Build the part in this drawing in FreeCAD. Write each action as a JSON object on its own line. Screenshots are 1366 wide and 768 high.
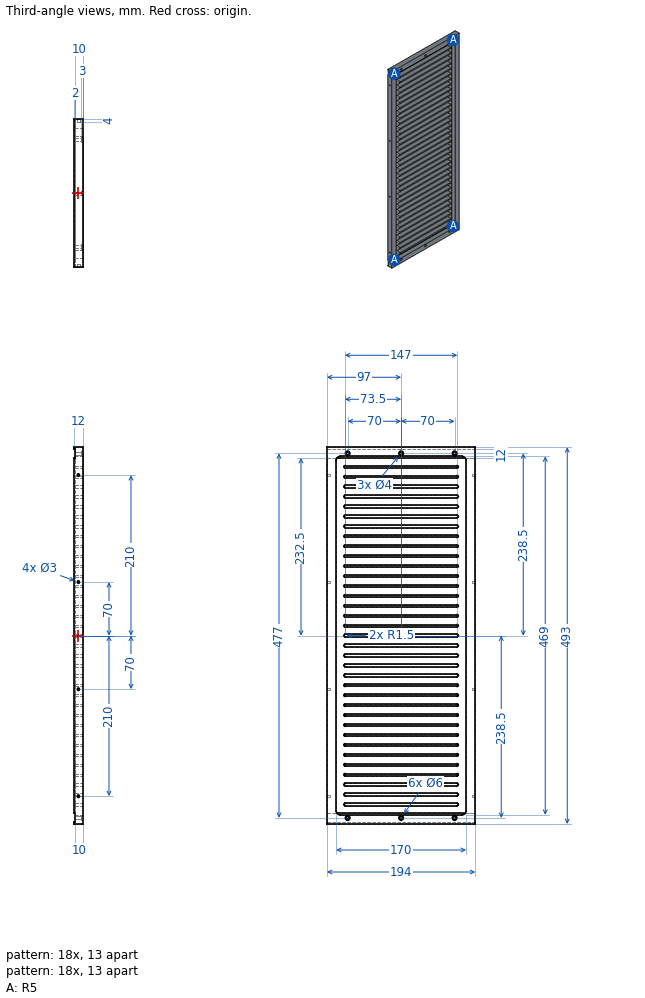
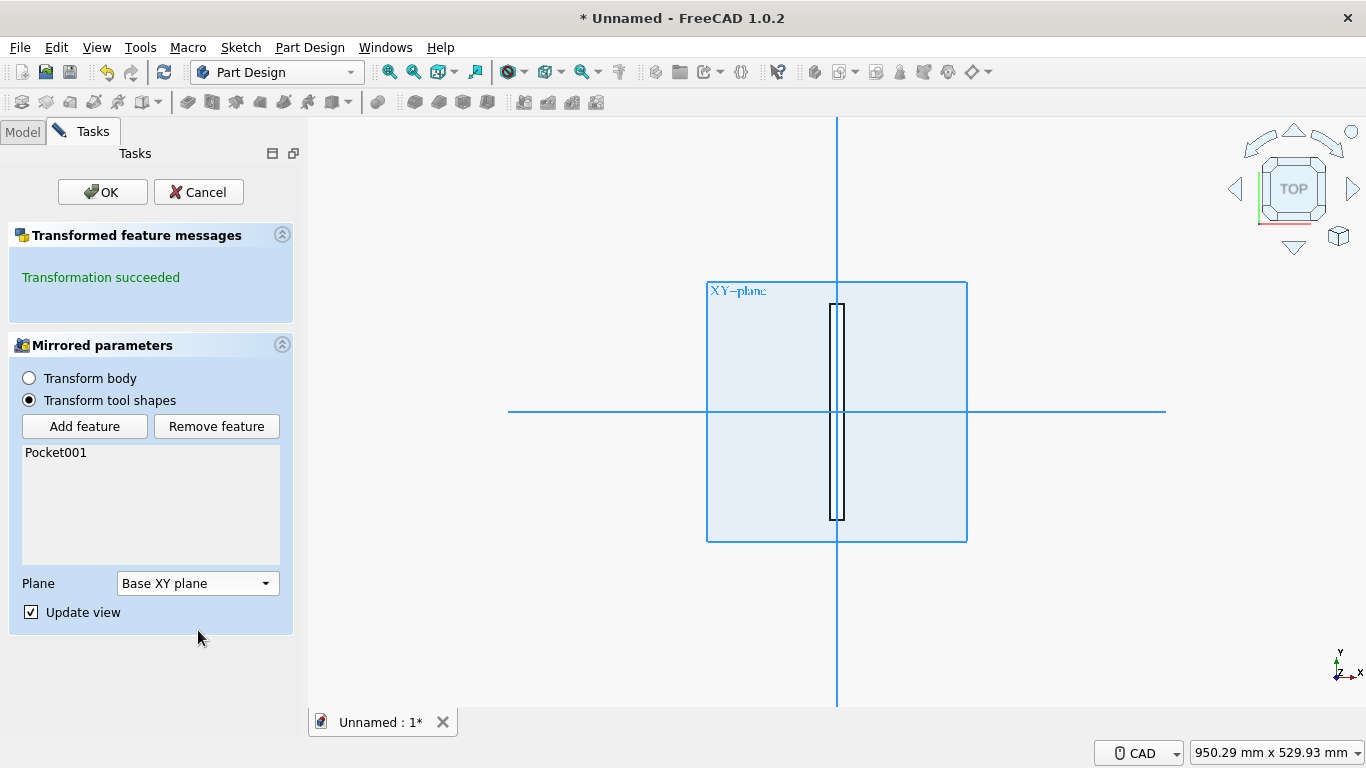
{"action": "left_click", "coordinate": [103, 192]}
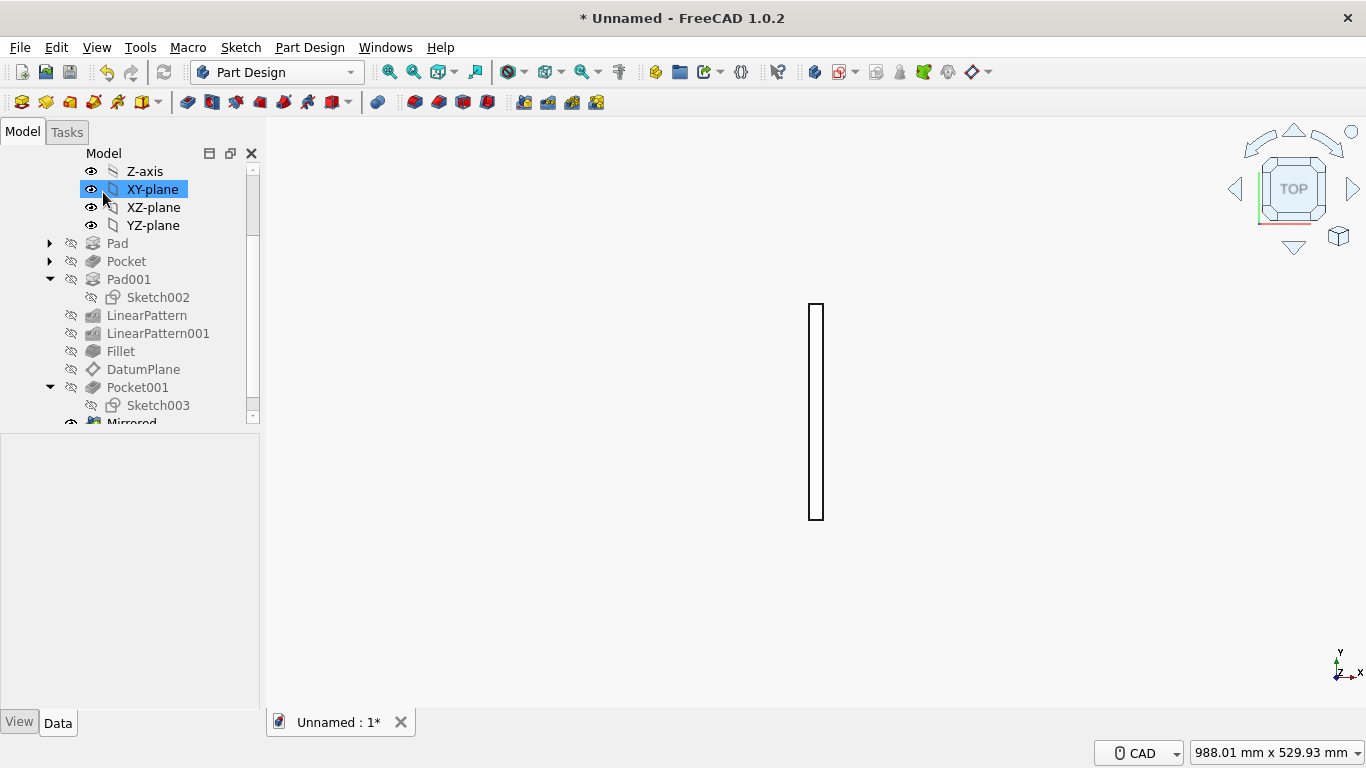
{"action": "left_click", "coordinate": [390, 72]}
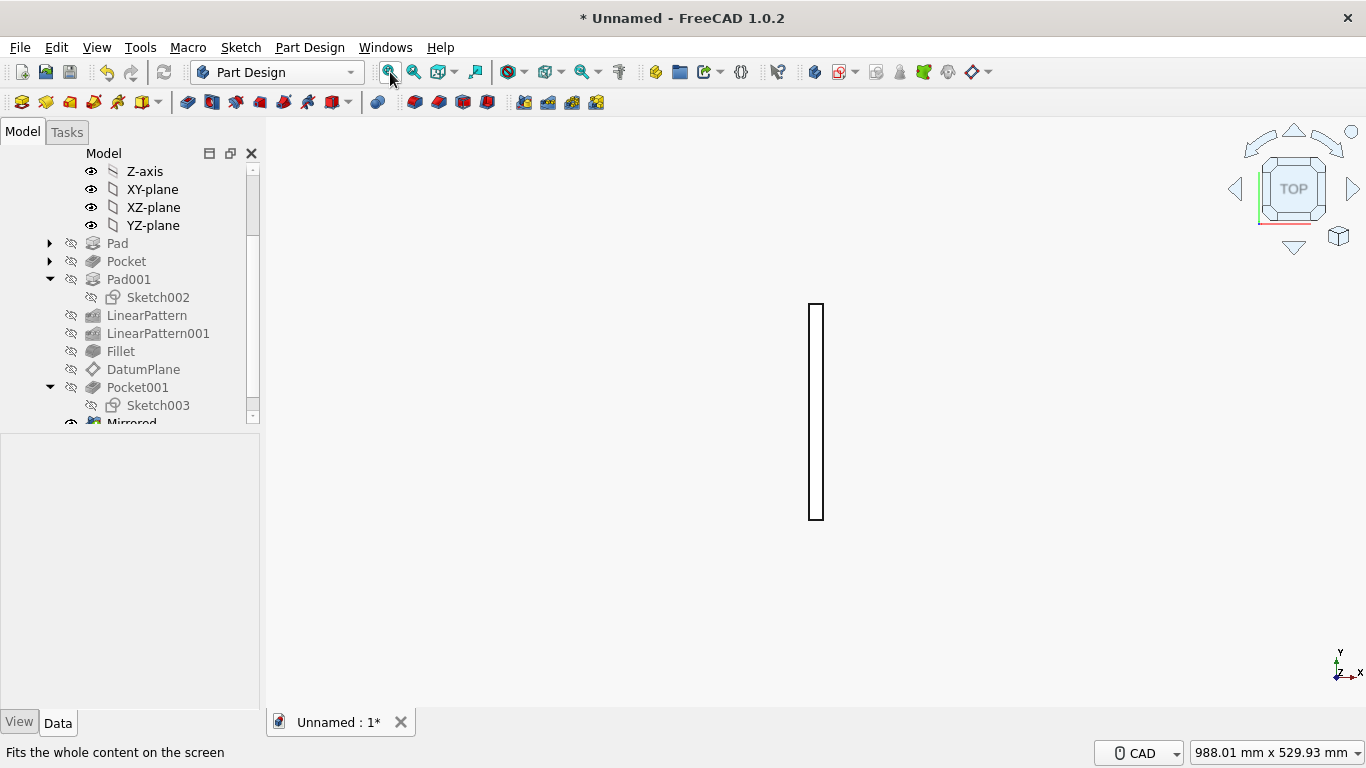
{"action": "key", "text": "6"}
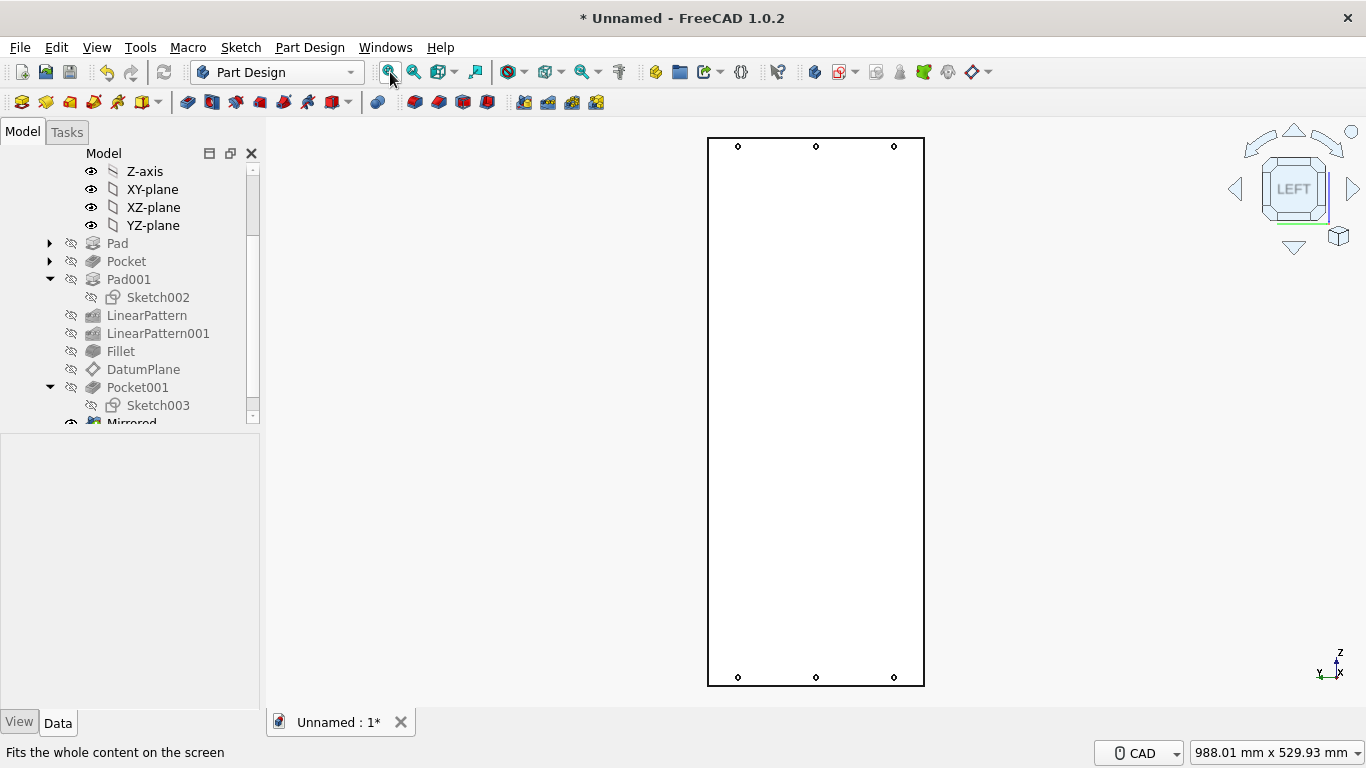
{"action": "left_click", "coordinate": [816, 489]}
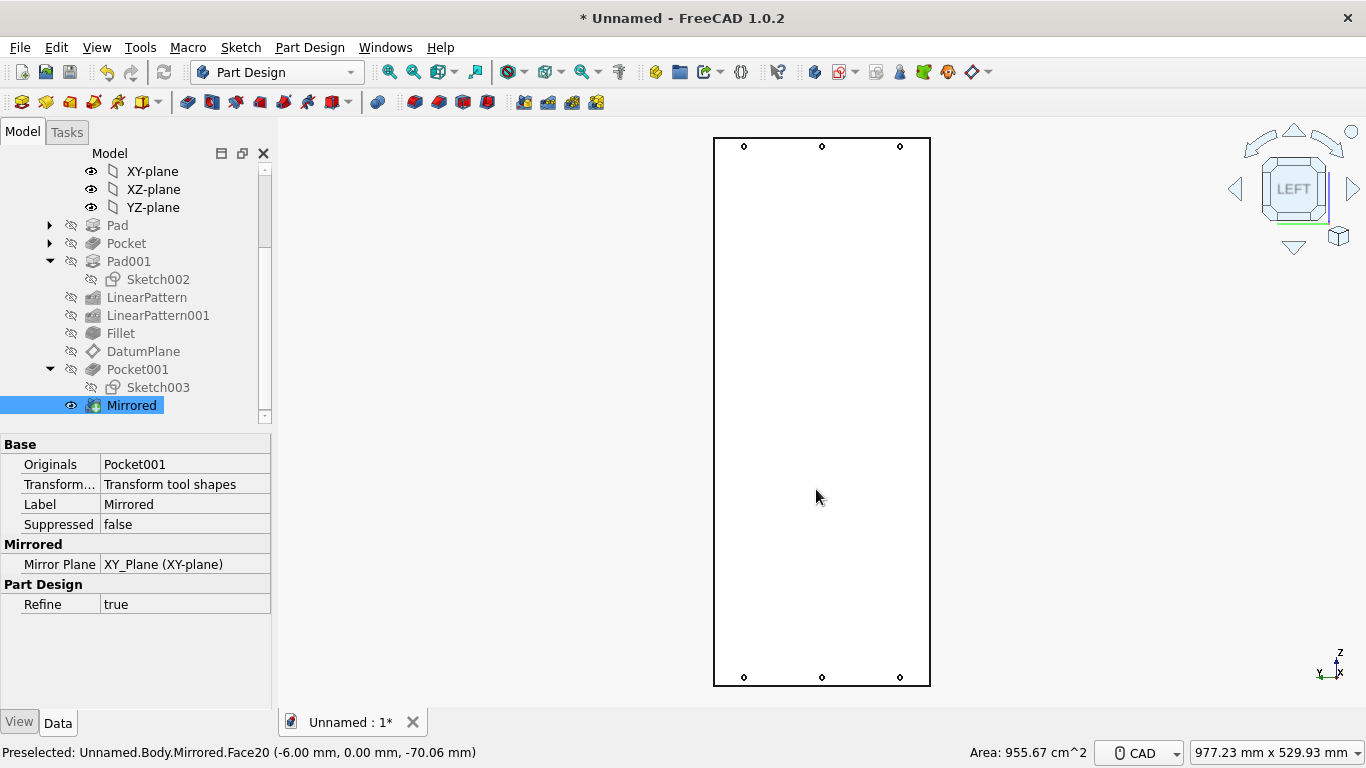
{"action": "left_click", "coordinate": [840, 72]}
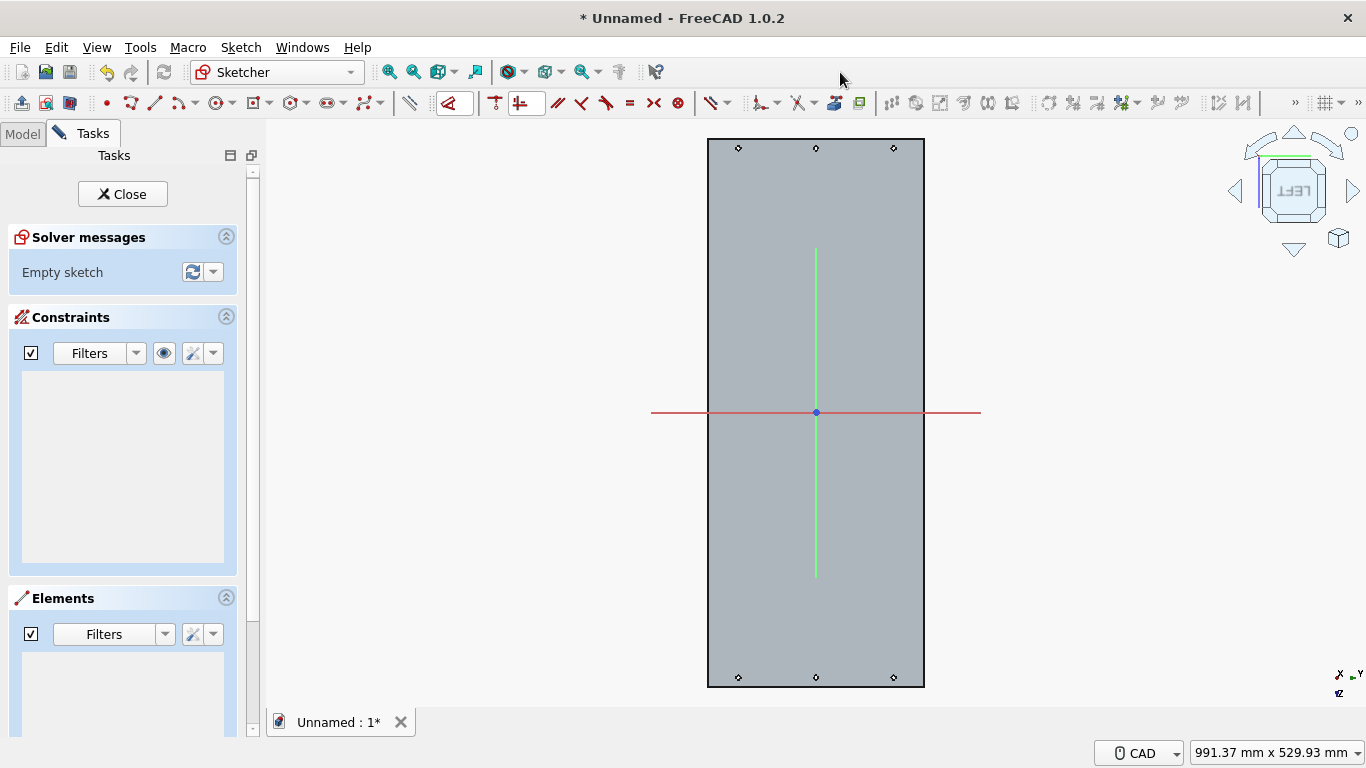
{"action": "scroll", "coordinate": [438, 147], "scroll_direction": "down", "scroll_amount": 1}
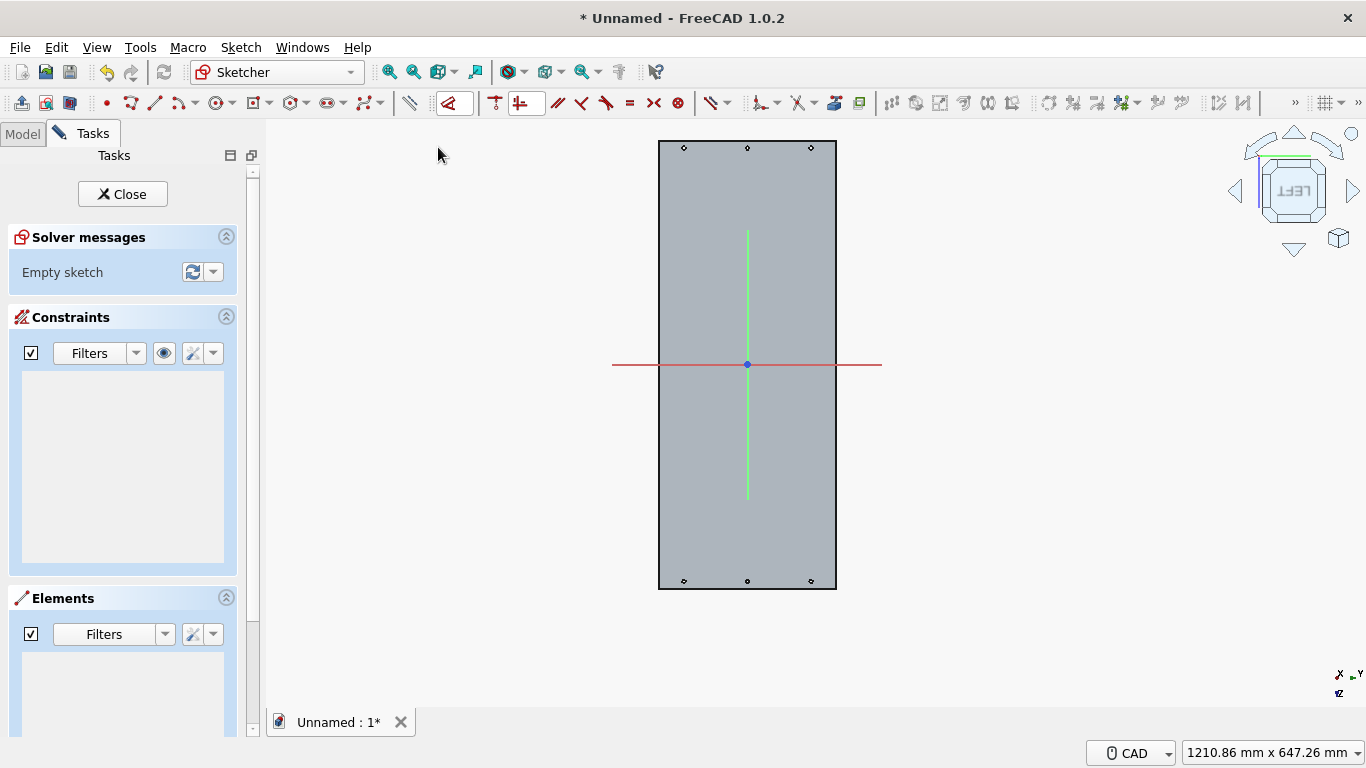
{"action": "scroll", "coordinate": [748, 552], "scroll_direction": "up", "scroll_amount": 3}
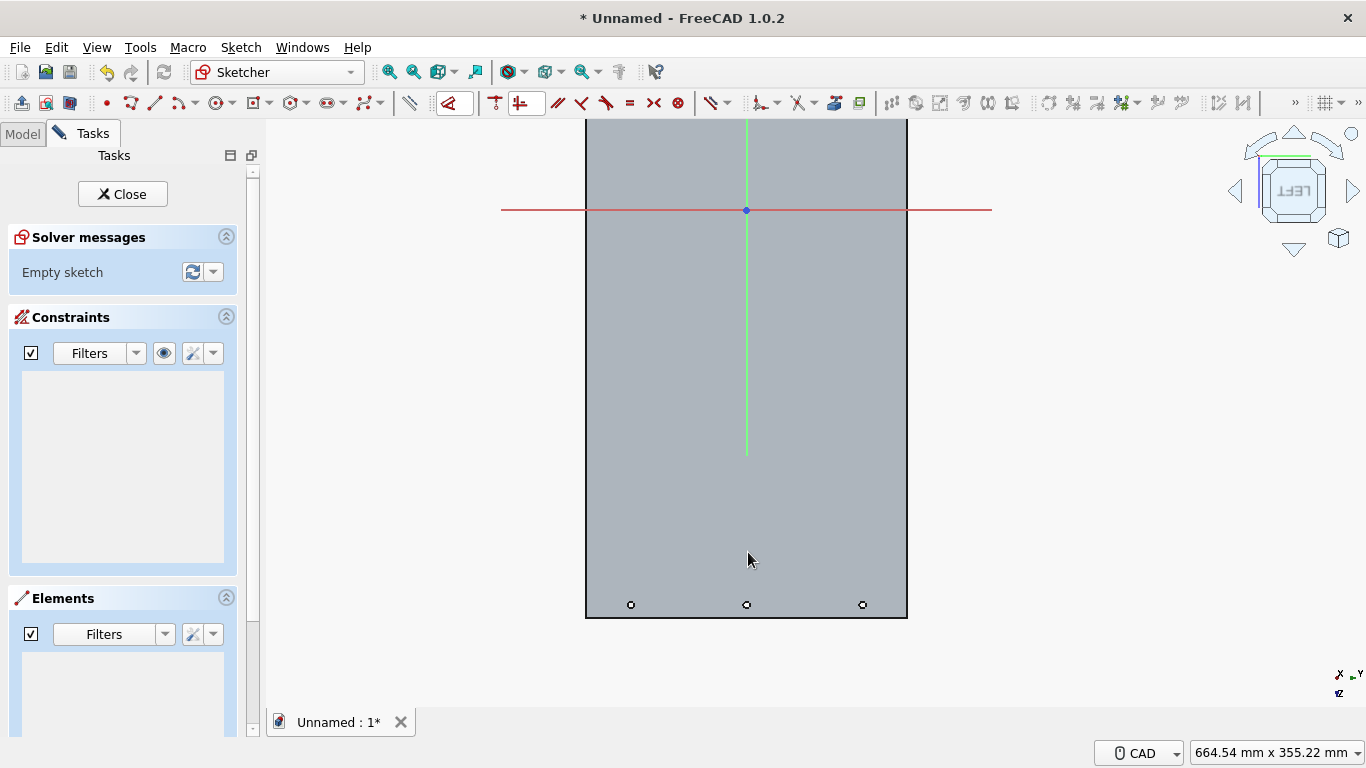
{"action": "key", "text": "g r"}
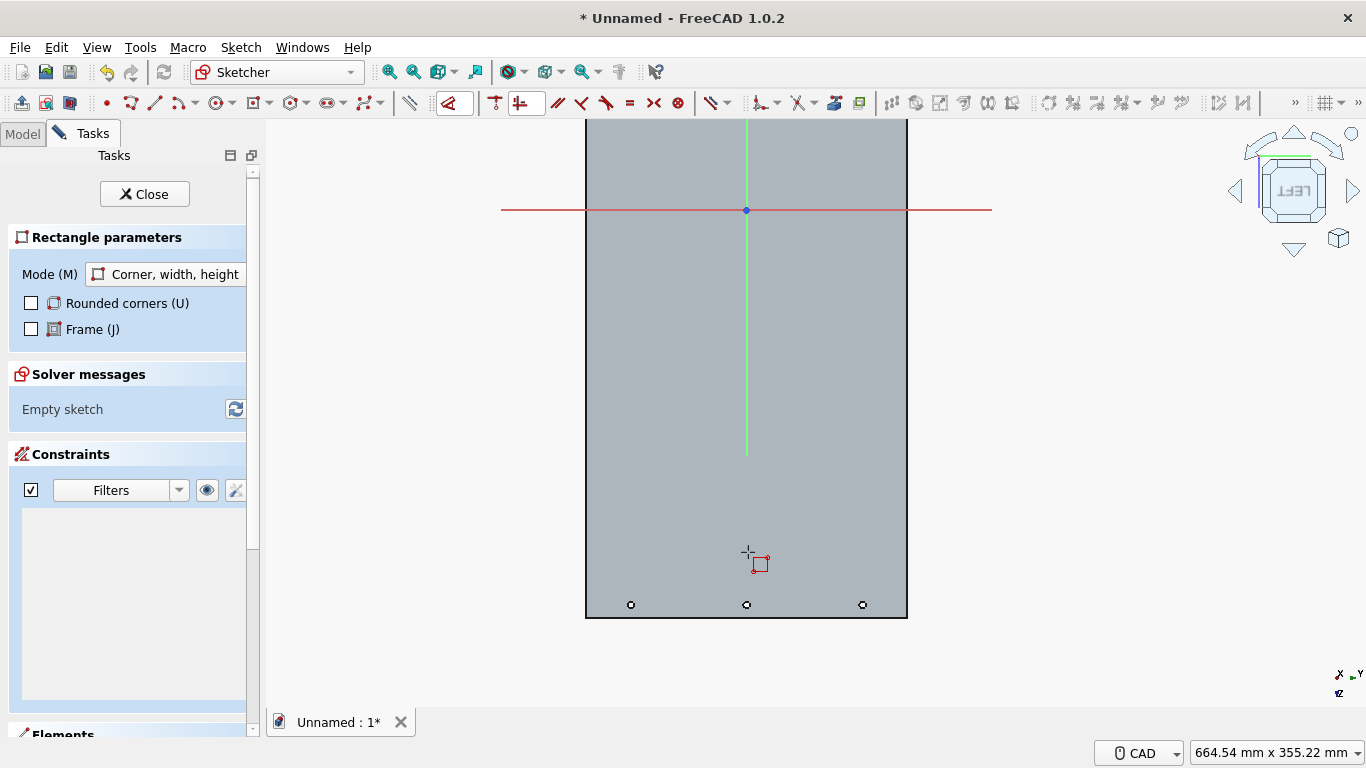
{"action": "left_click", "coordinate": [586, 595]}
{"action": "mouse_move", "coordinate": [907, 615]}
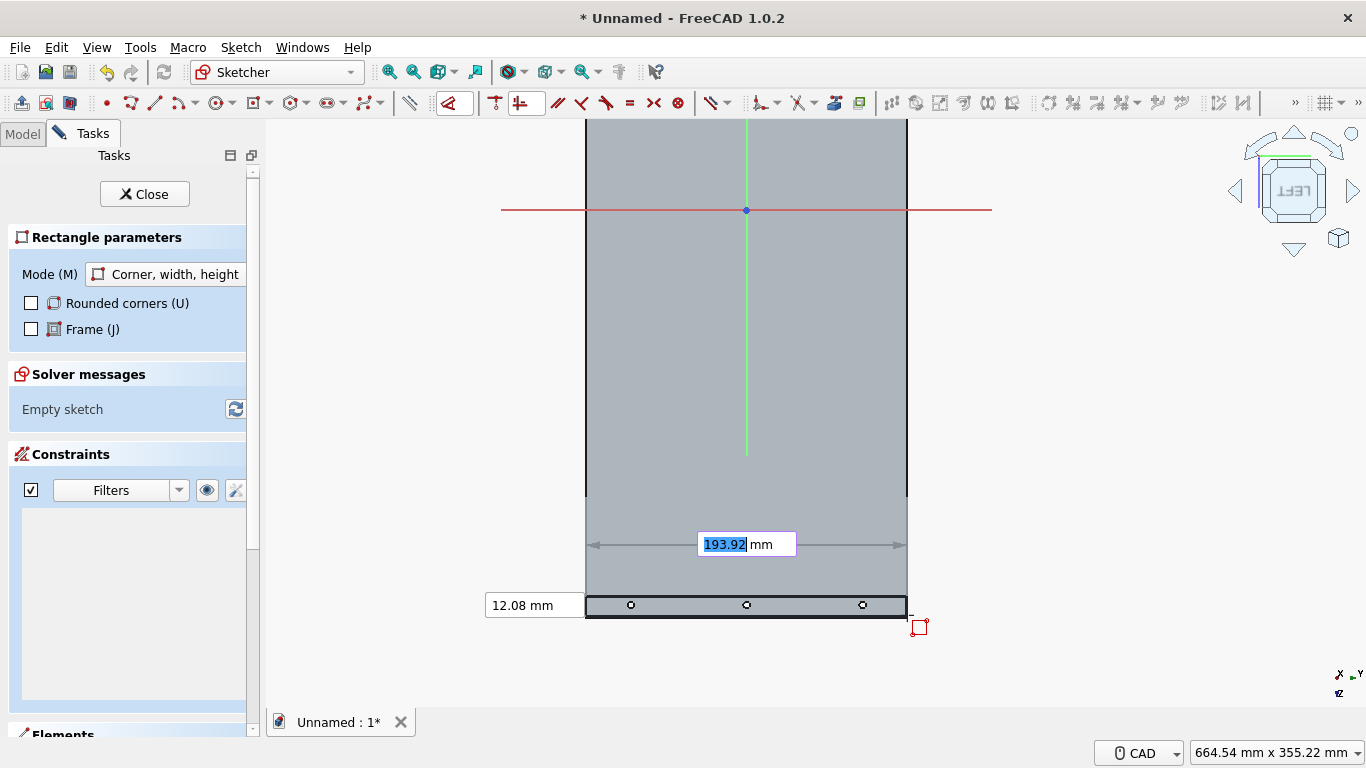
{"action": "type", "text": "194"}
{"action": "key", "text": "Tab"}
{"action": "type", "text": "12"}
{"action": "key", "text": "Return"}
{"action": "key", "text": "Escape"}